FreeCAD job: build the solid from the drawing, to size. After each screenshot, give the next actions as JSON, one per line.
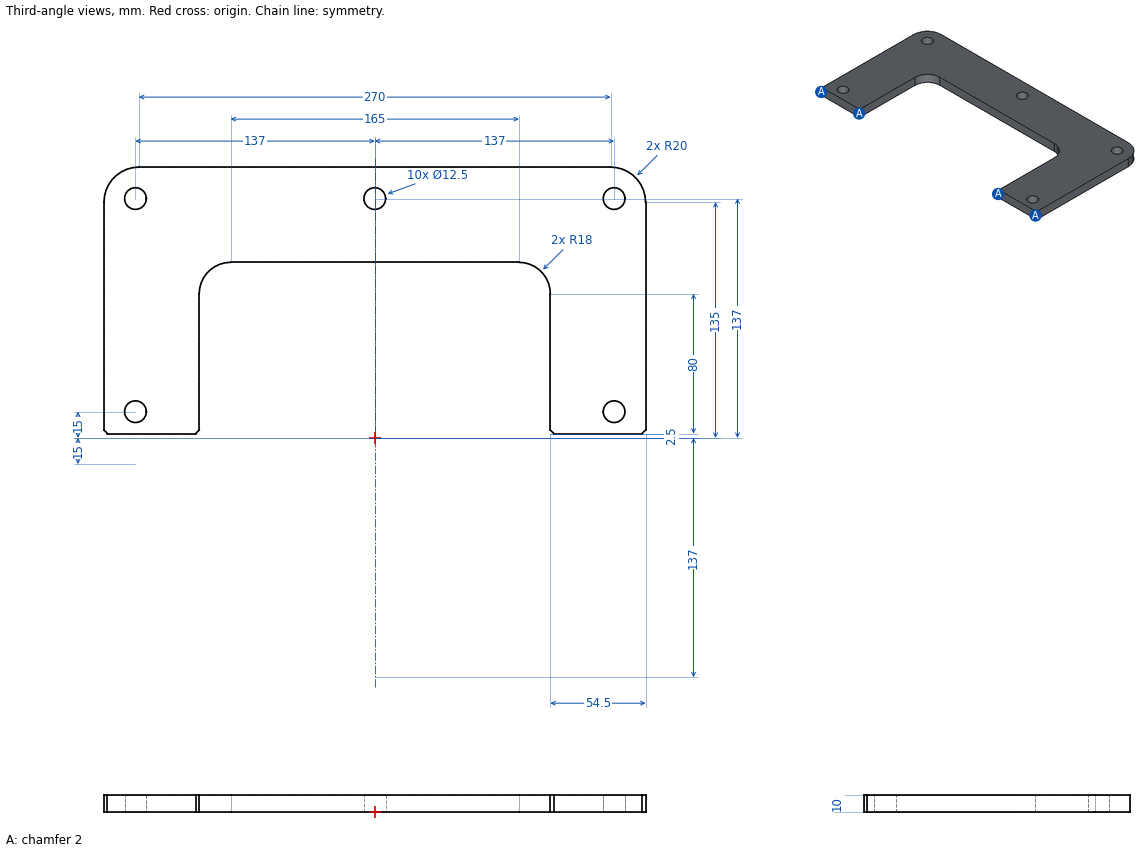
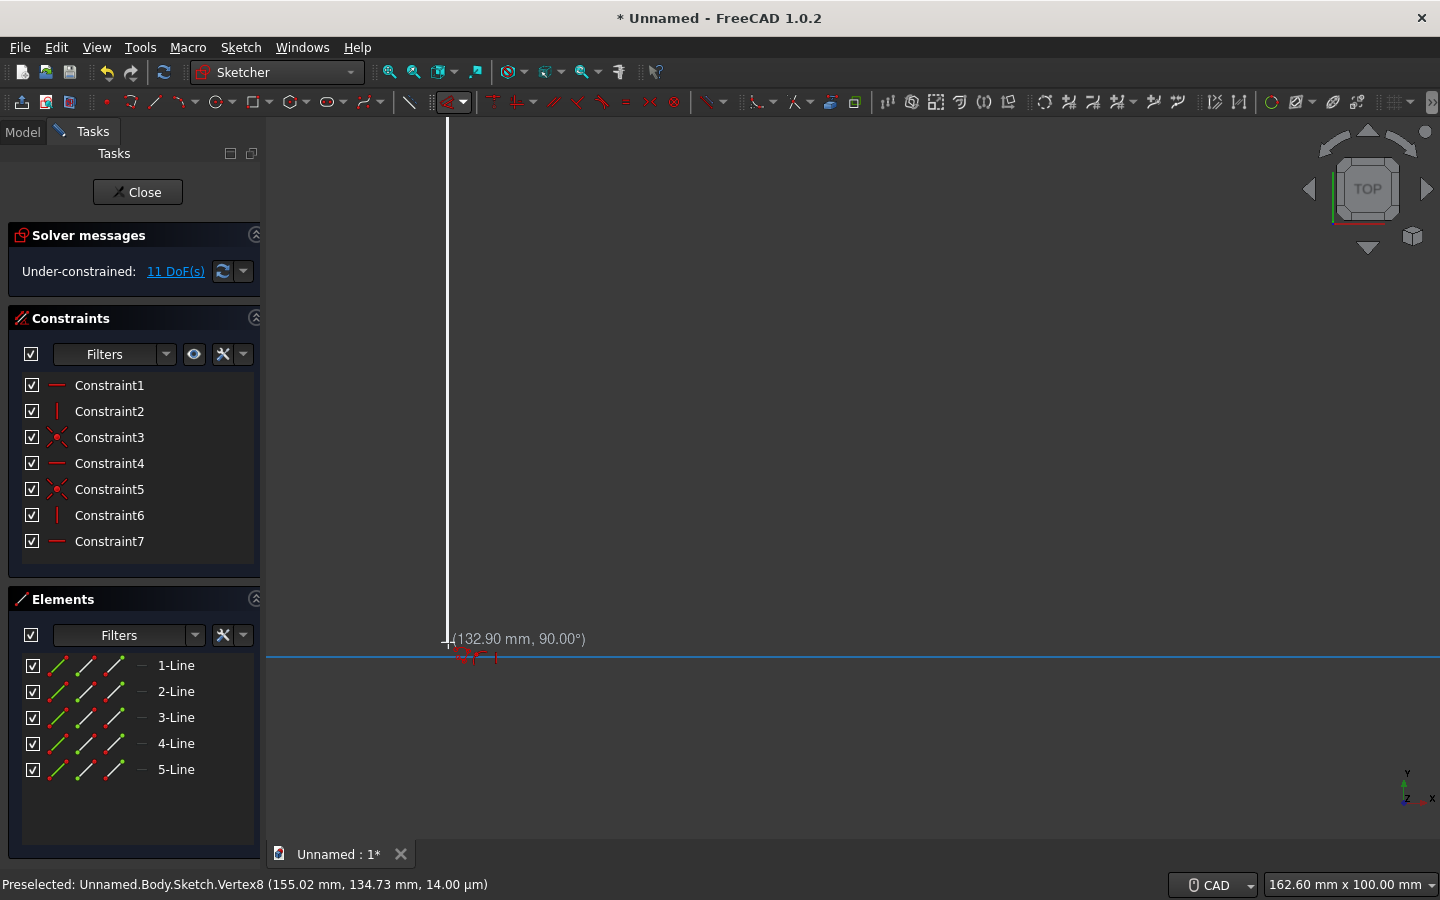
{"action": "left_click", "coordinate": [448, 639]}
{"action": "left_click", "coordinate": [840, 639]}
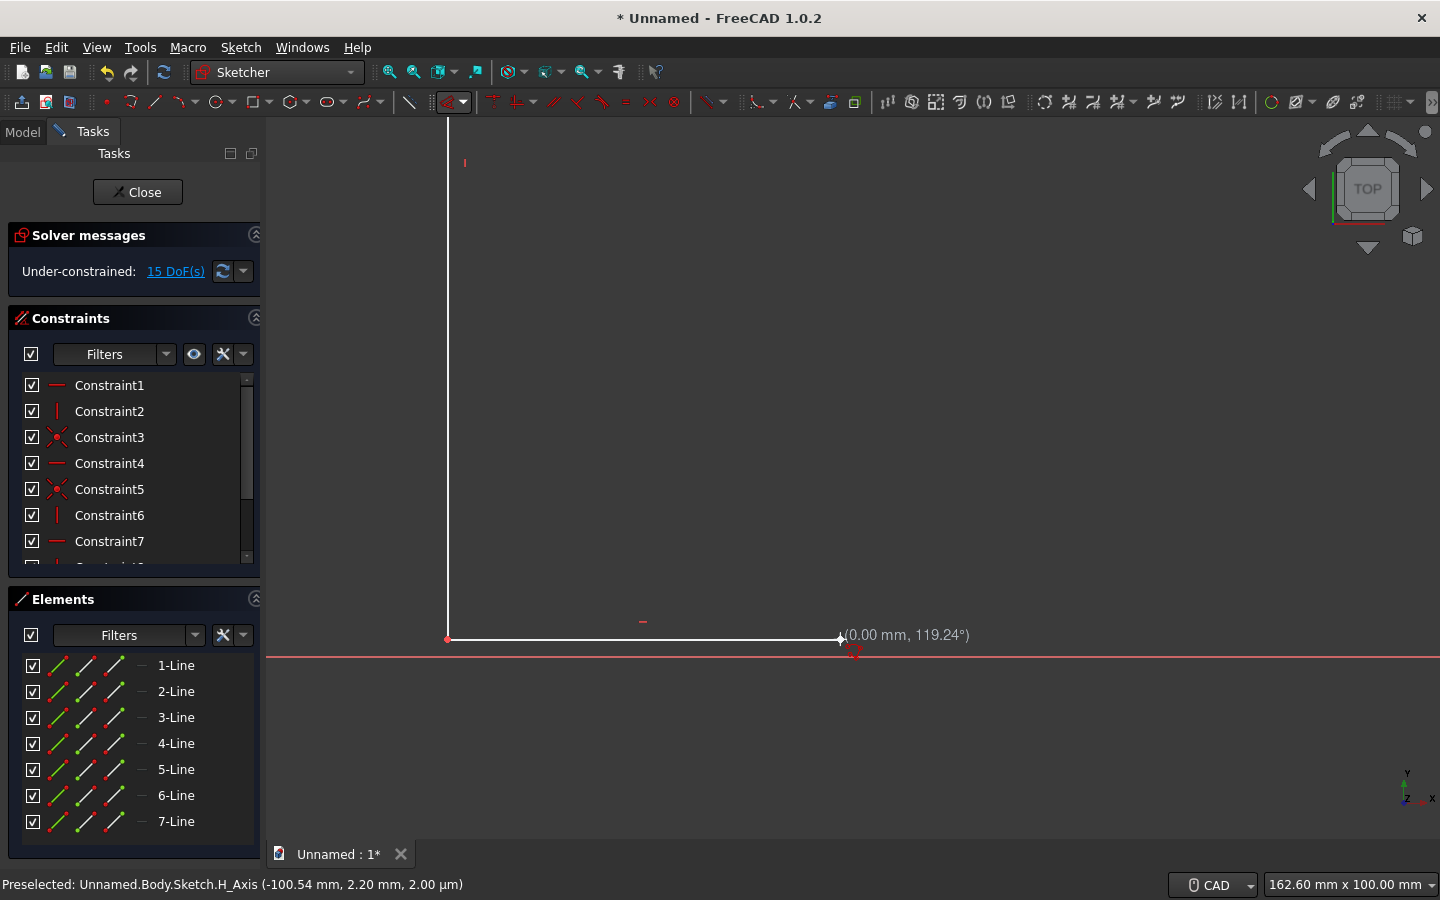
{"action": "scroll", "coordinate": [448, 642], "scroll_direction": "down", "scroll_amount": 6}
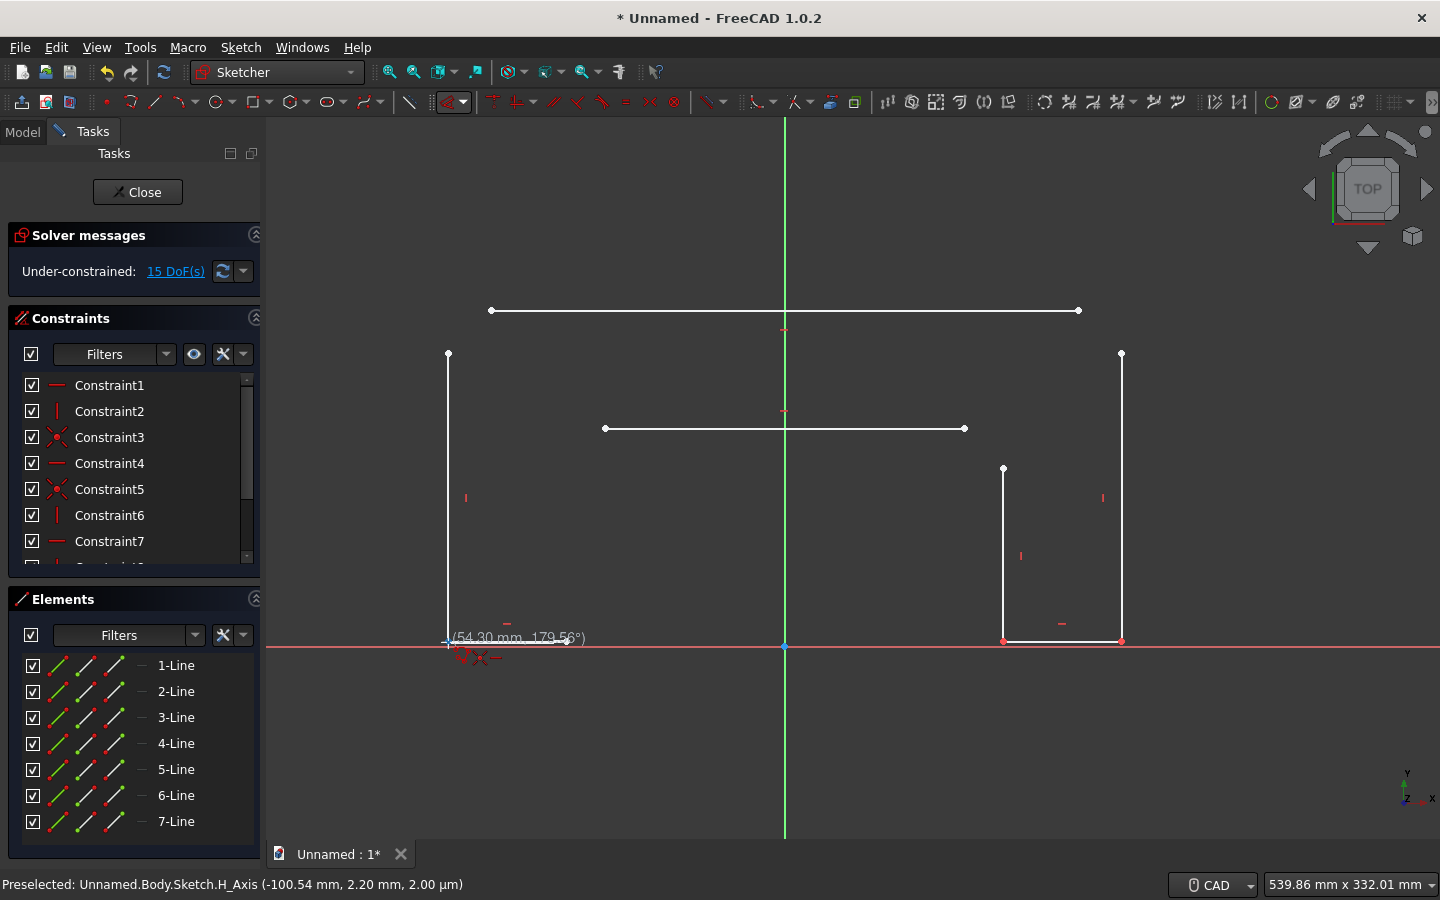
{"action": "left_click", "coordinate": [566, 468]}
{"action": "right_click", "coordinate": [566, 468]}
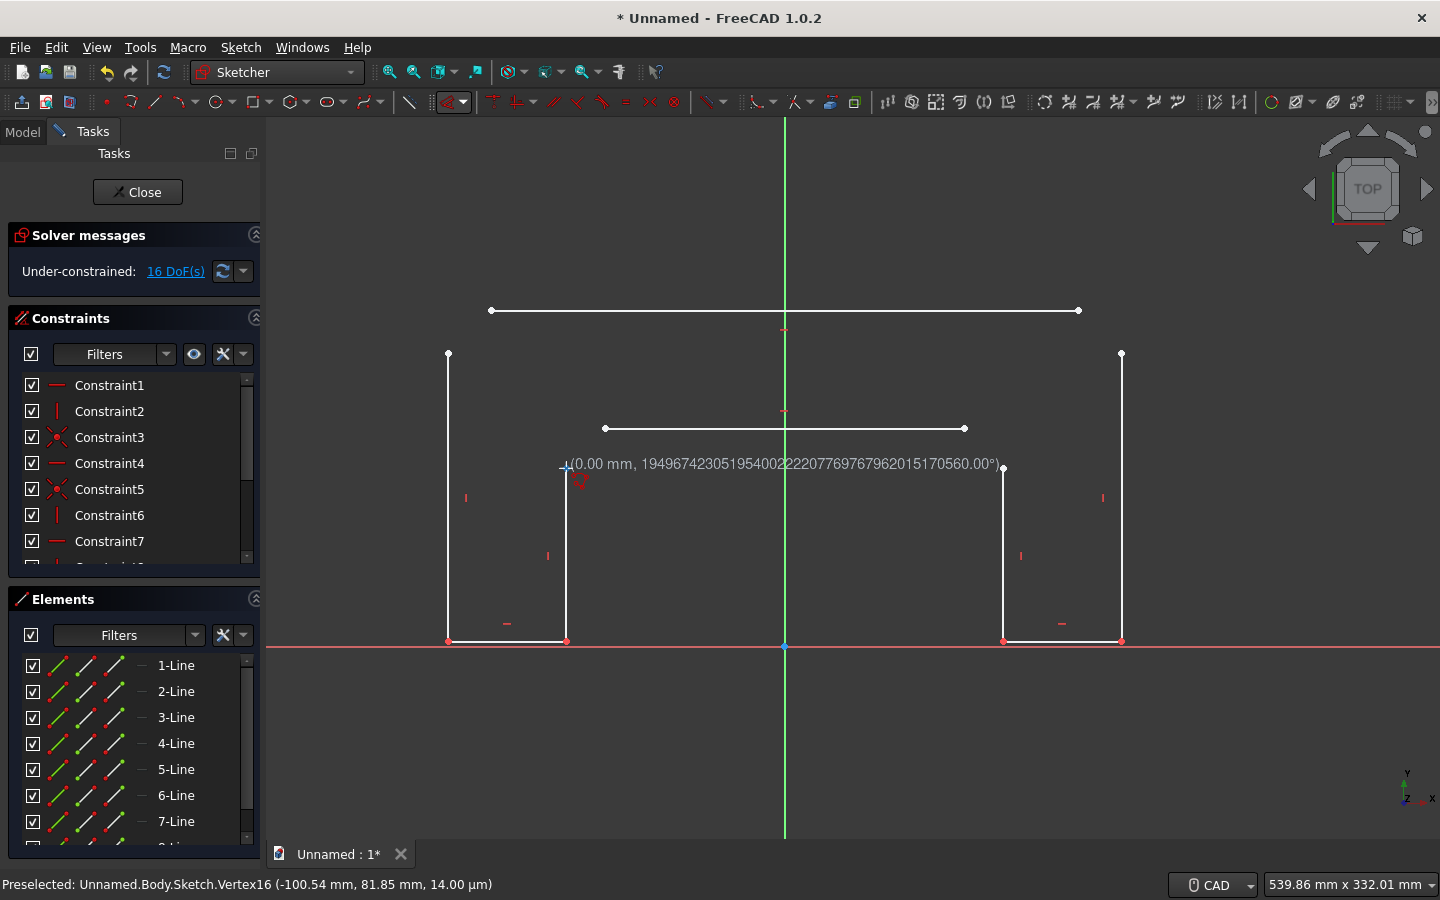
{"action": "left_click", "coordinate": [180, 102]}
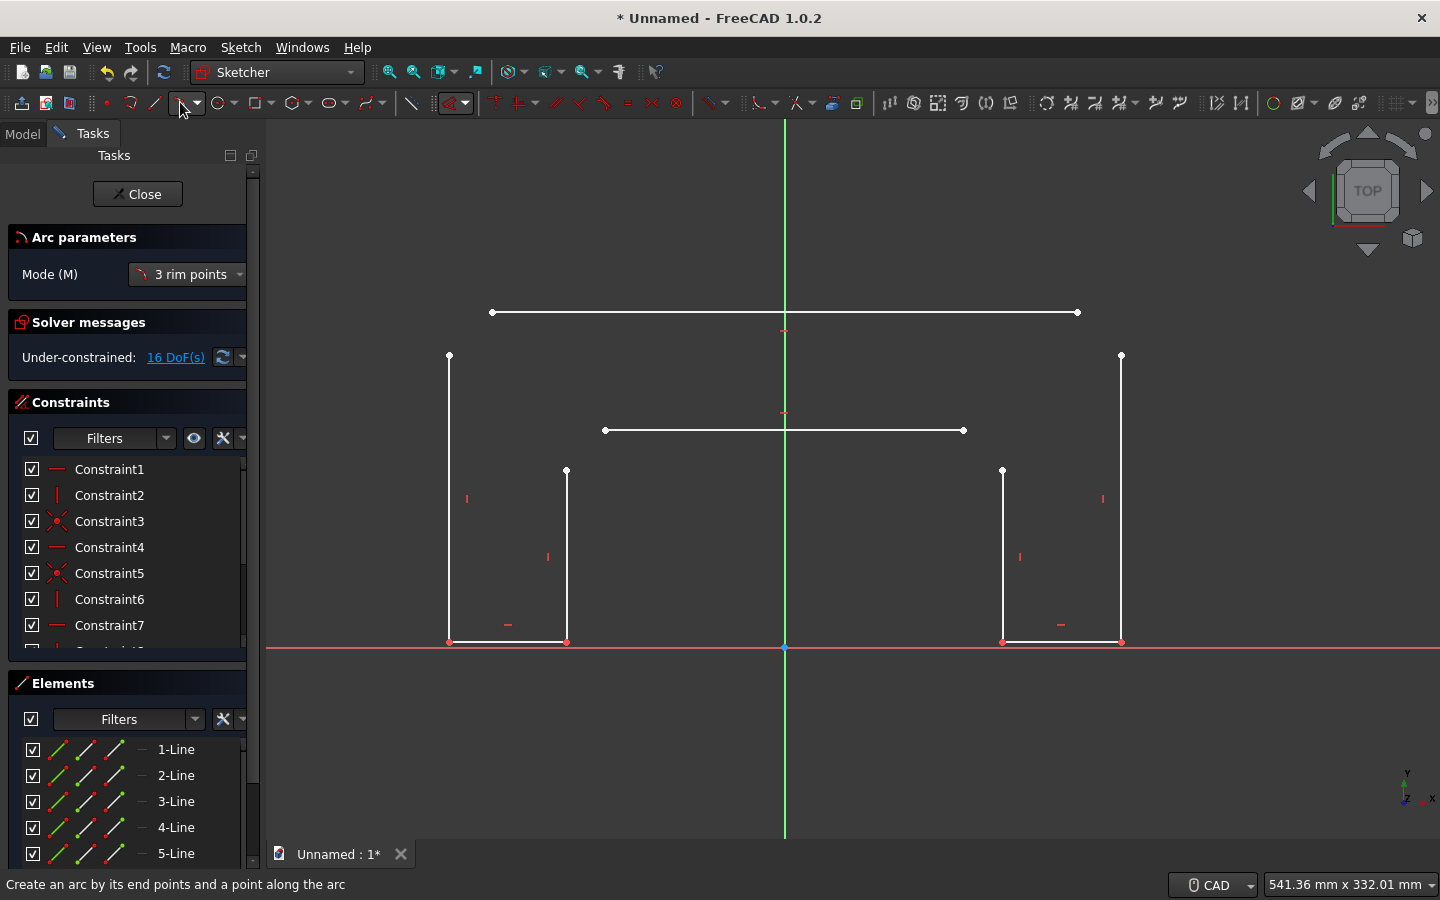
{"action": "left_click", "coordinate": [964, 430]}
{"action": "left_click", "coordinate": [1003, 470]}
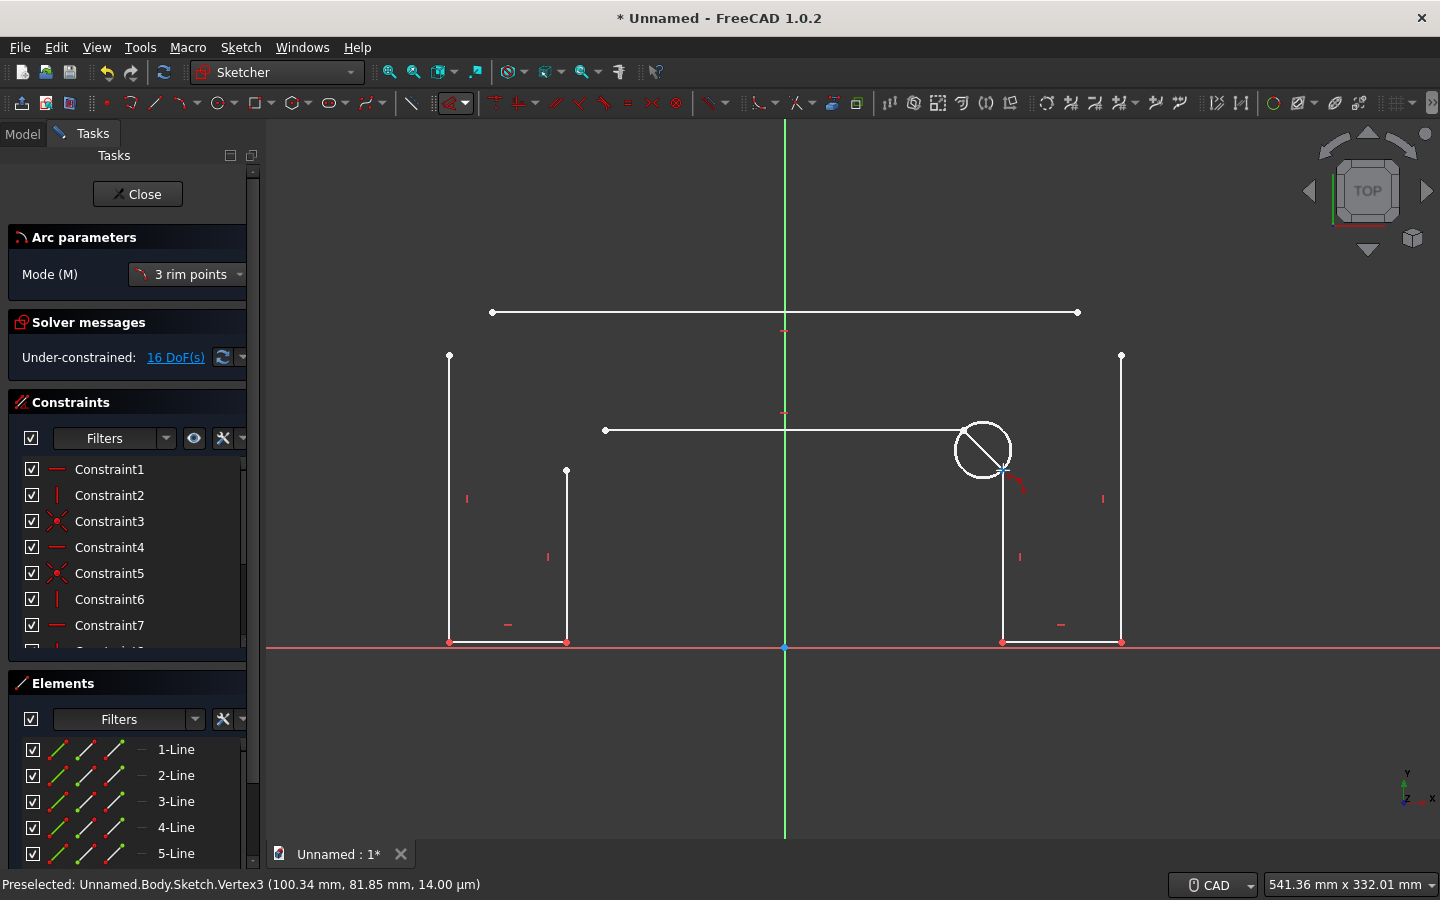
{"action": "scroll", "coordinate": [992, 441], "scroll_direction": "up", "scroll_amount": 2}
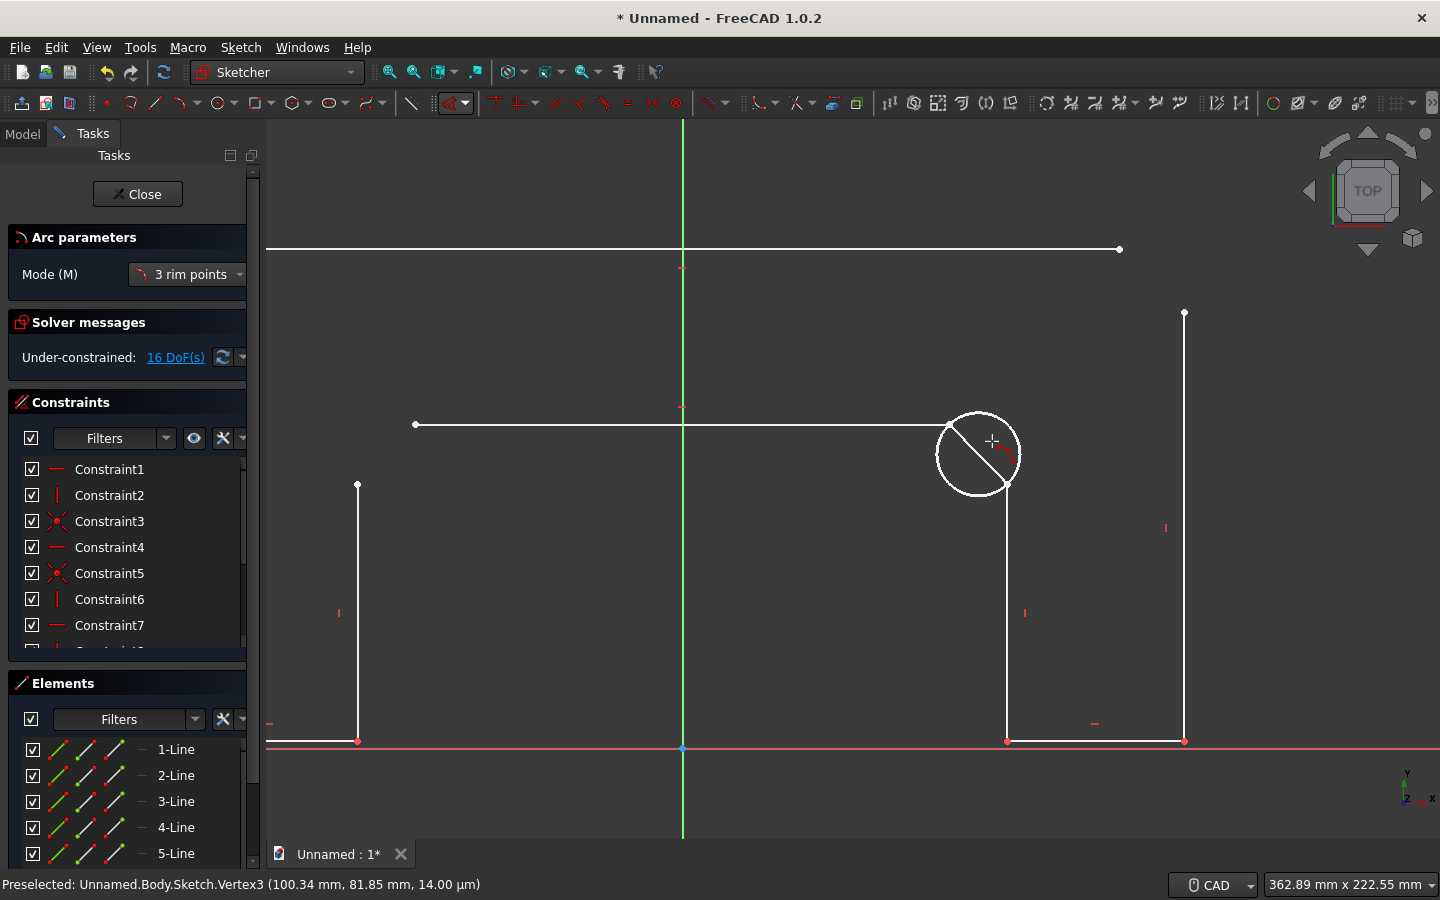
{"action": "left_click", "coordinate": [991, 441]}